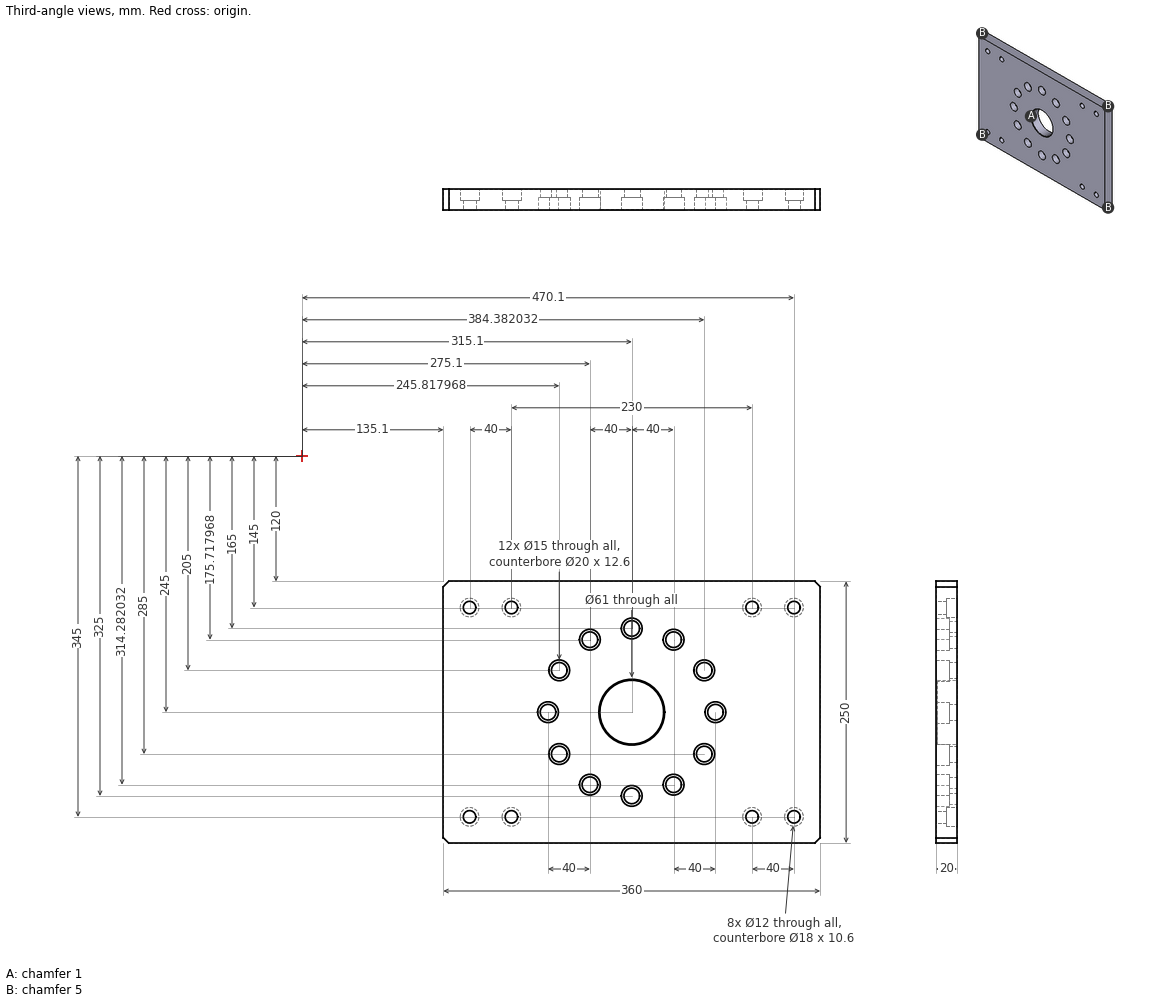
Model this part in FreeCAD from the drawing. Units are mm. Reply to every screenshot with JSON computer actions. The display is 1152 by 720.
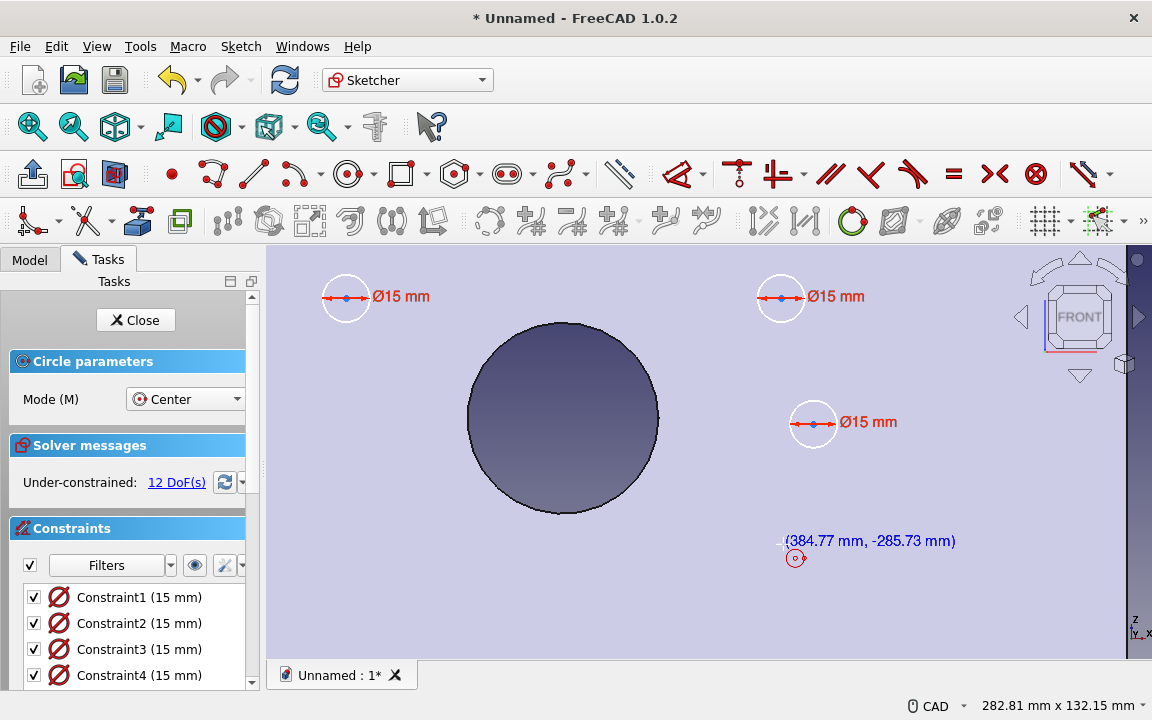
{"action": "scroll", "coordinate": [783, 544], "scroll_direction": "down", "scroll_amount": 7}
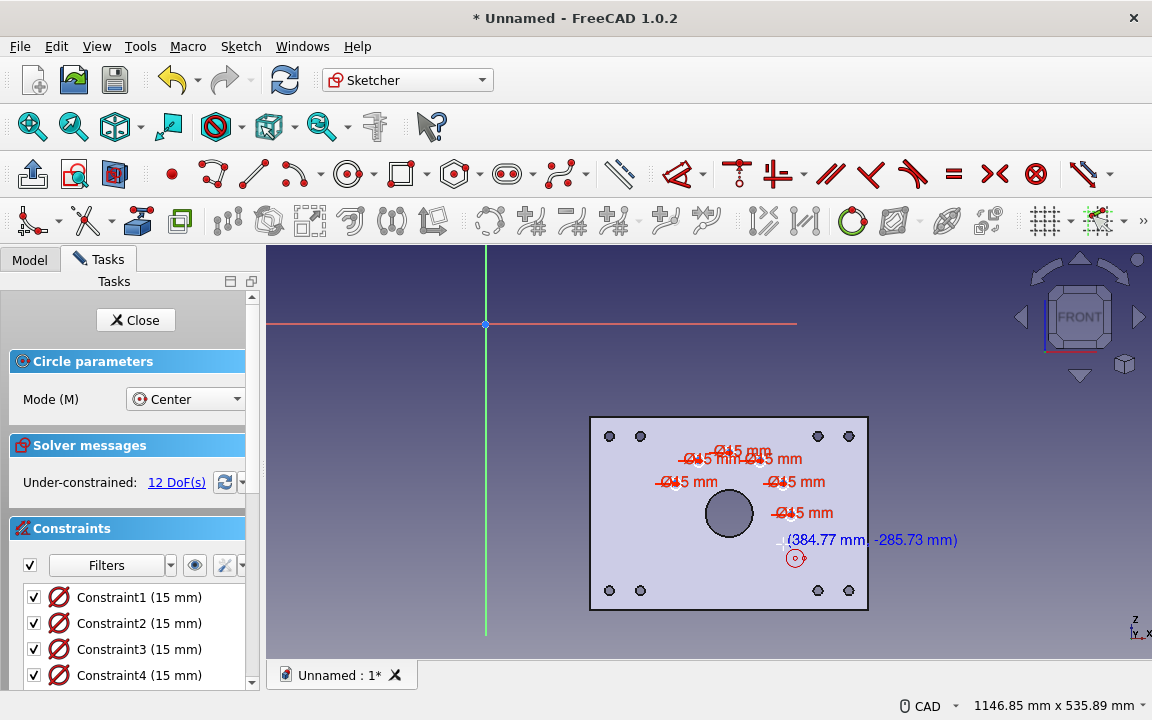
{"action": "left_click", "coordinate": [783, 544]}
{"action": "mouse_move", "coordinate": [787, 540]}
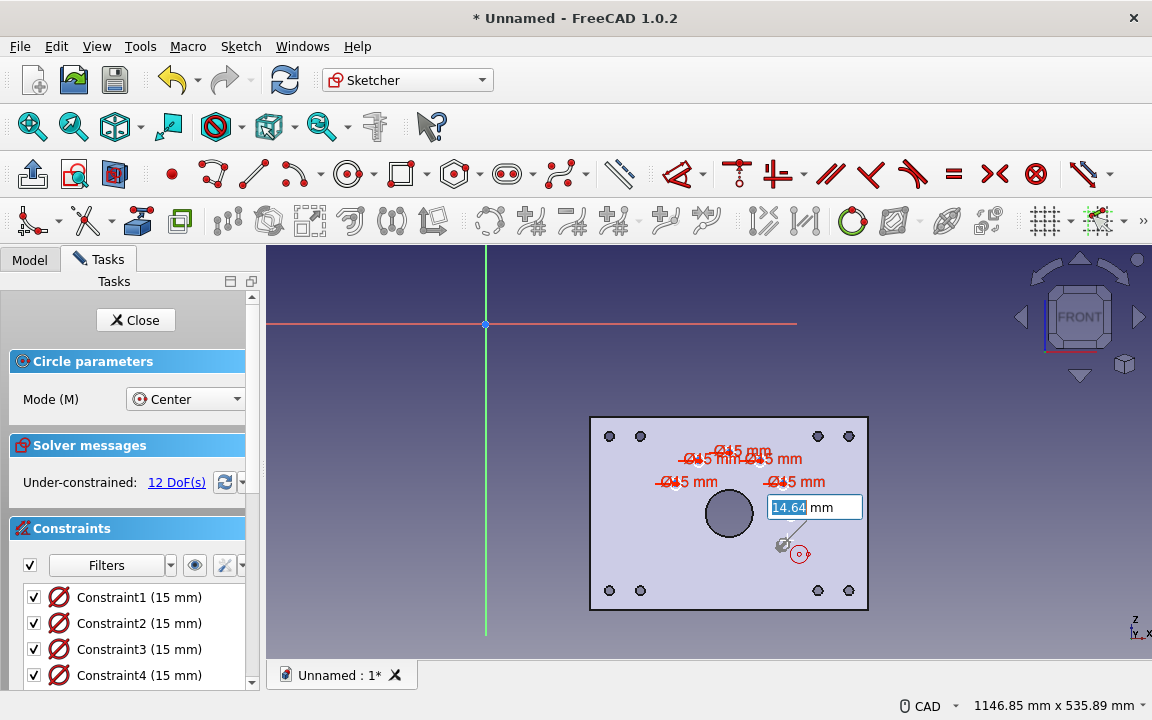
{"action": "type", "text": "15"}
{"action": "key", "text": "Return"}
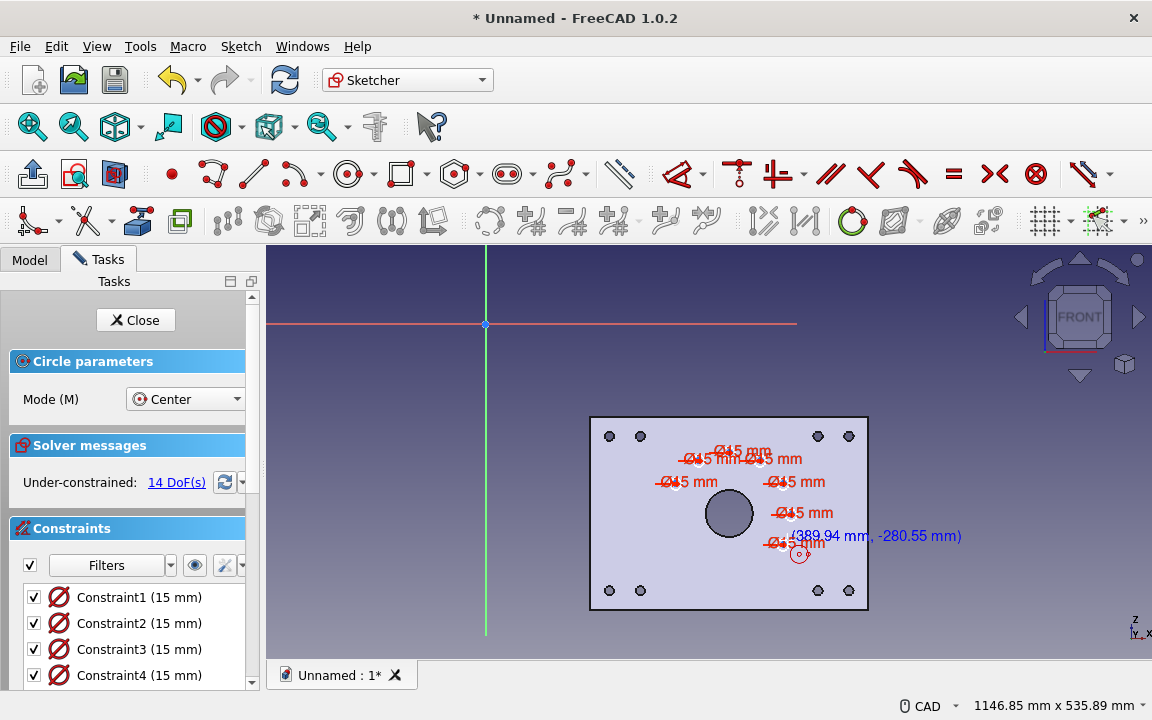
{"action": "scroll", "coordinate": [760, 567], "scroll_direction": "up", "scroll_amount": 7}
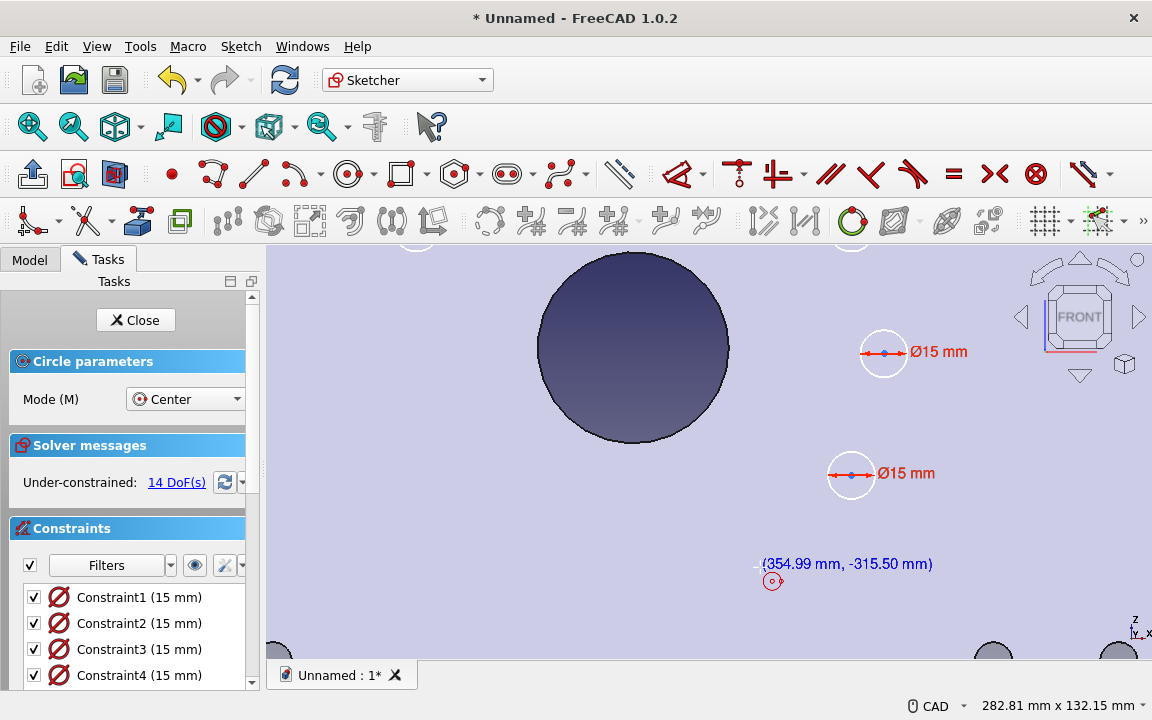
{"action": "scroll", "coordinate": [760, 567], "scroll_direction": "down", "scroll_amount": 7}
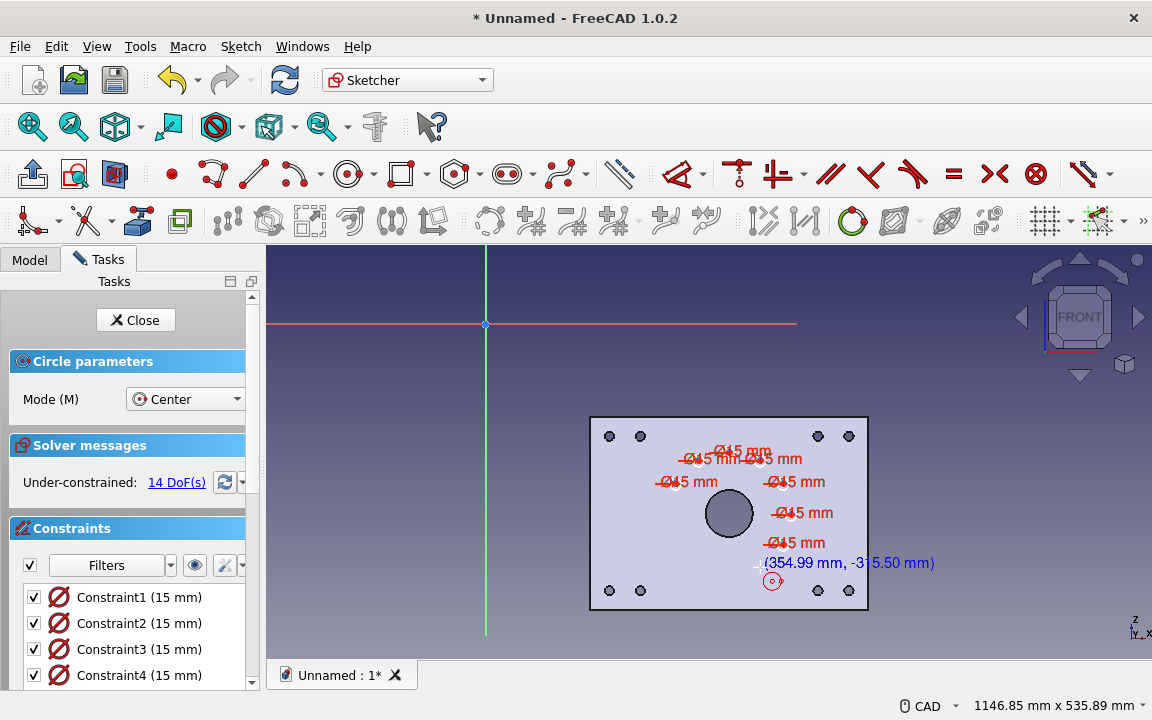
{"action": "left_click", "coordinate": [760, 567]}
{"action": "mouse_move", "coordinate": [764, 563]}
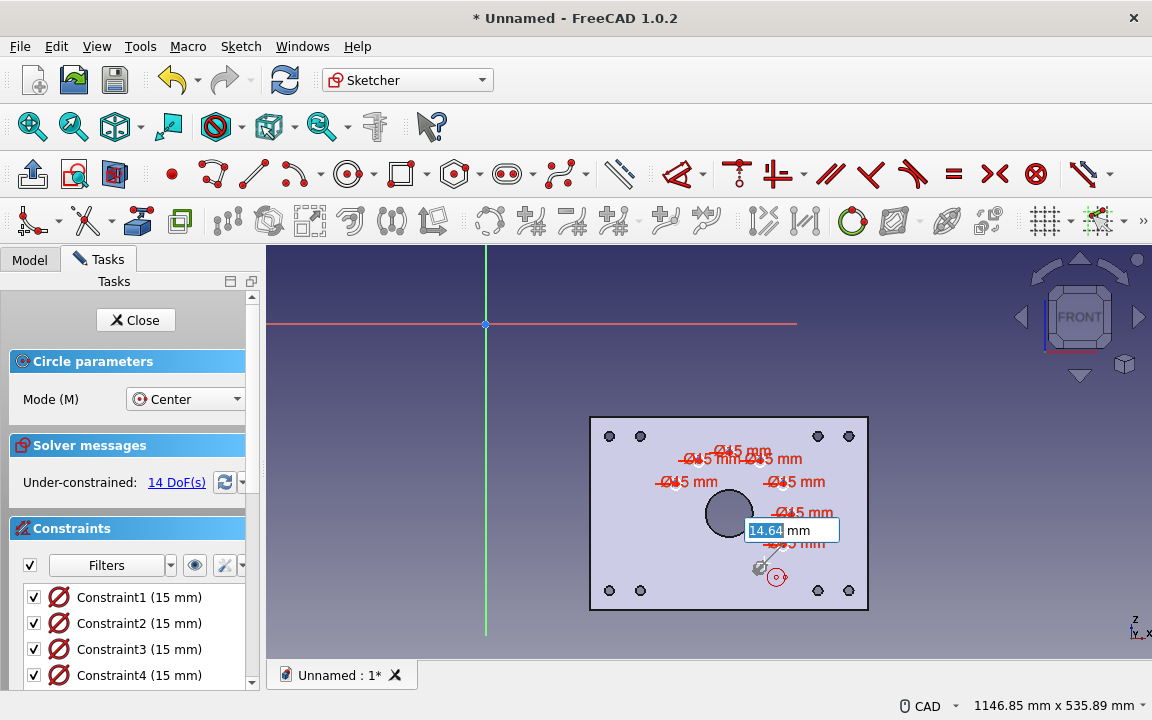
{"action": "type", "text": "15"}
{"action": "key", "text": "Return"}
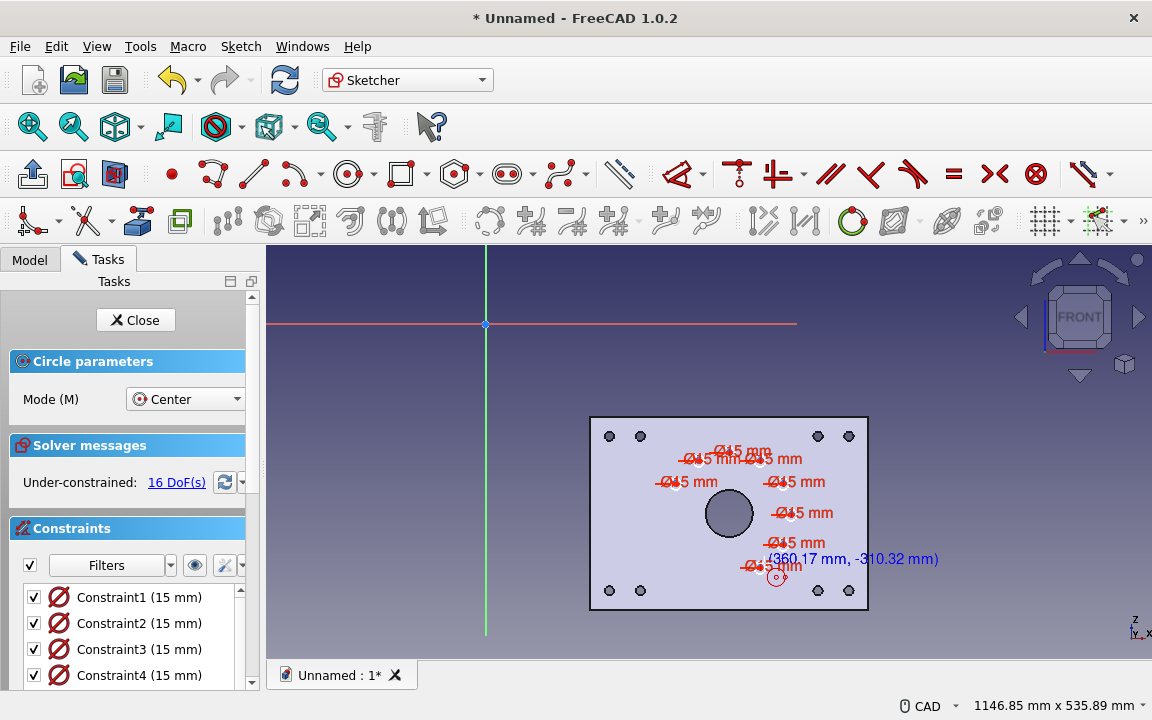
{"action": "scroll", "coordinate": [729, 575], "scroll_direction": "up", "scroll_amount": 7}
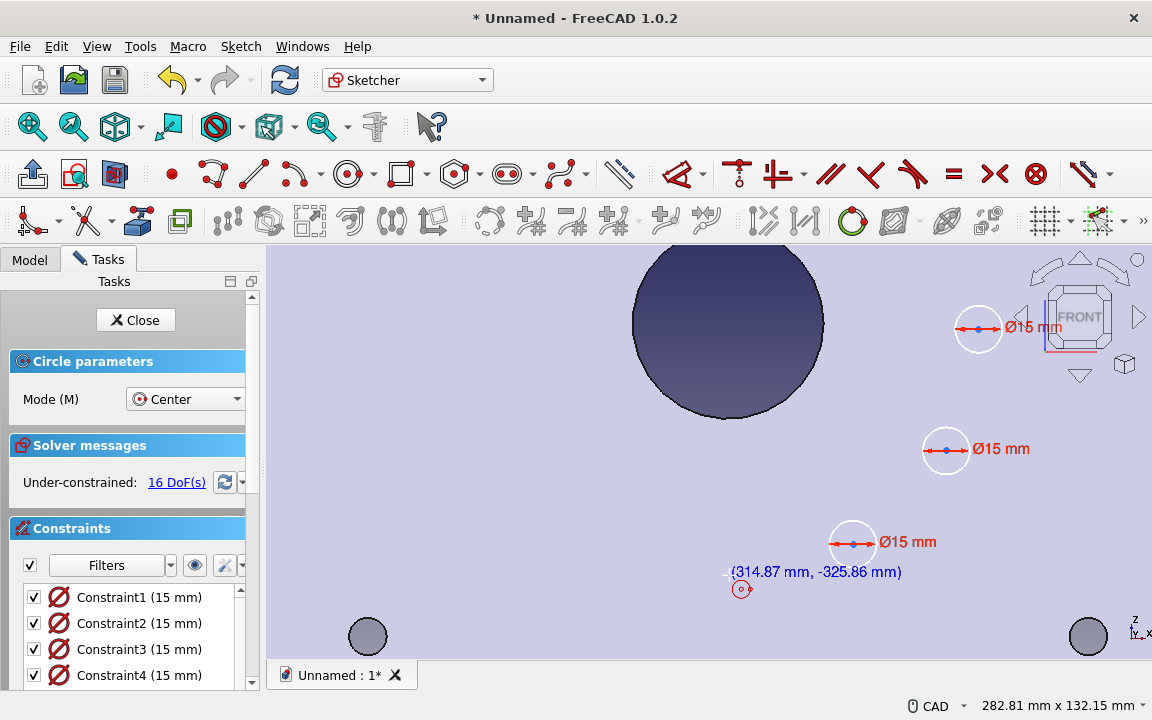
{"action": "scroll", "coordinate": [729, 575], "scroll_direction": "down", "scroll_amount": 7}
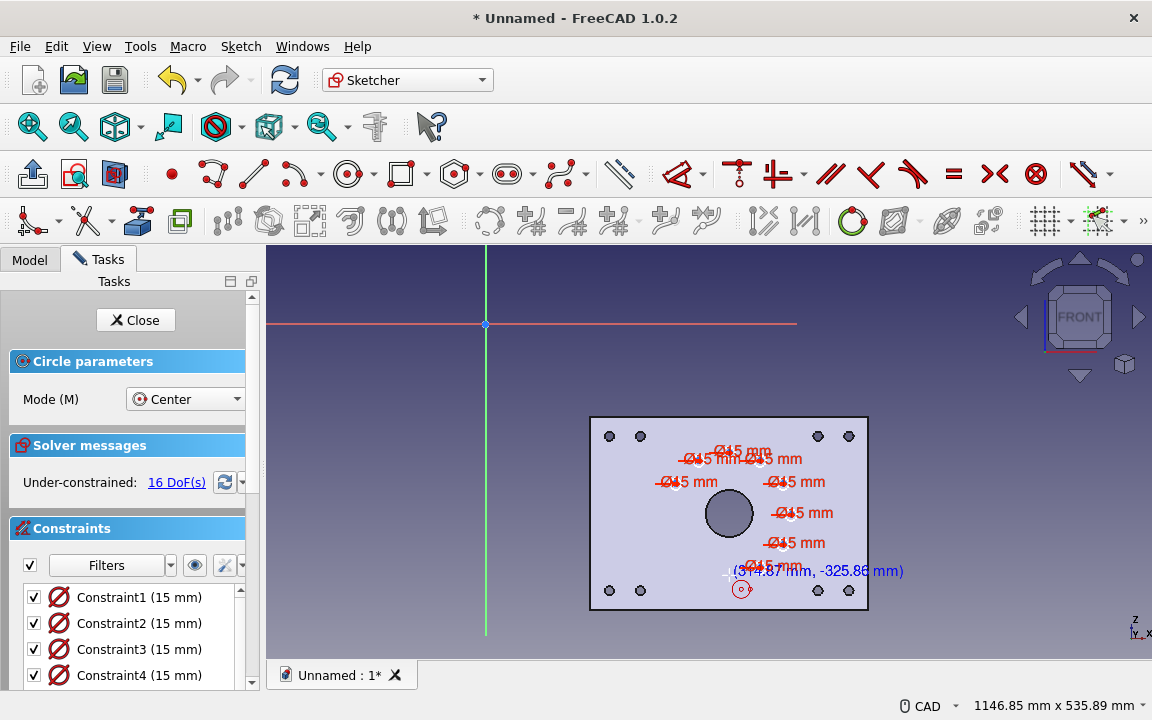
{"action": "left_click", "coordinate": [729, 575]}
{"action": "mouse_move", "coordinate": [733, 571]}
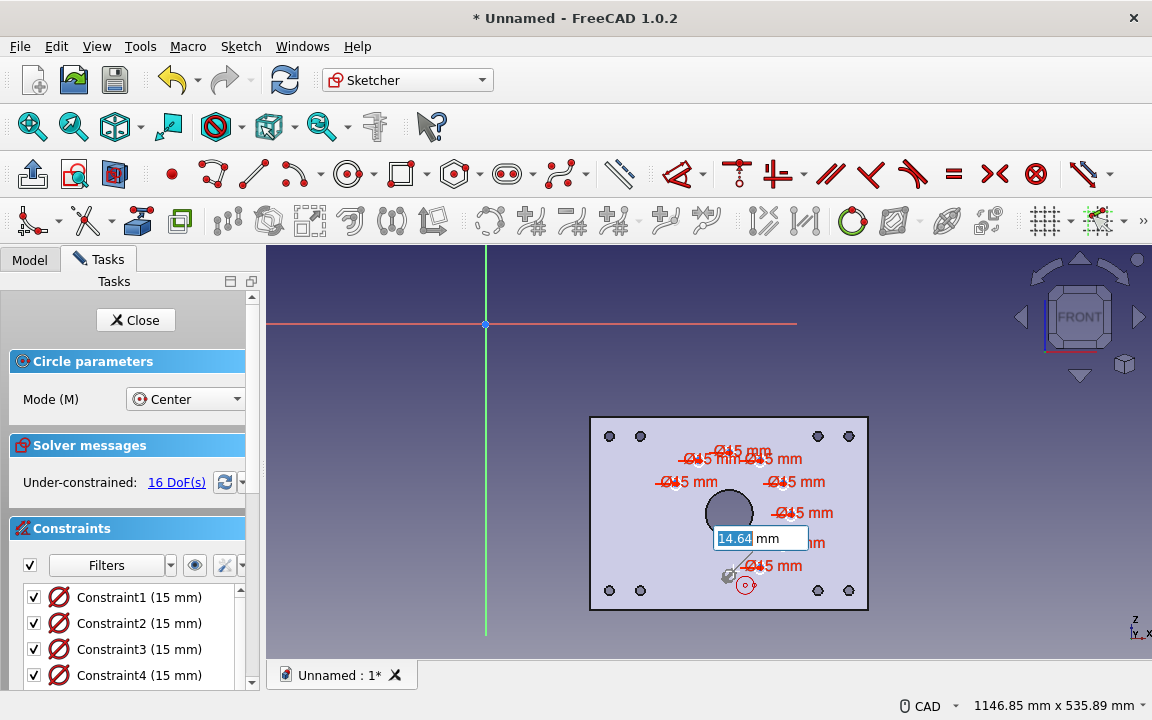
{"action": "type", "text": "15"}
{"action": "key", "text": "Return"}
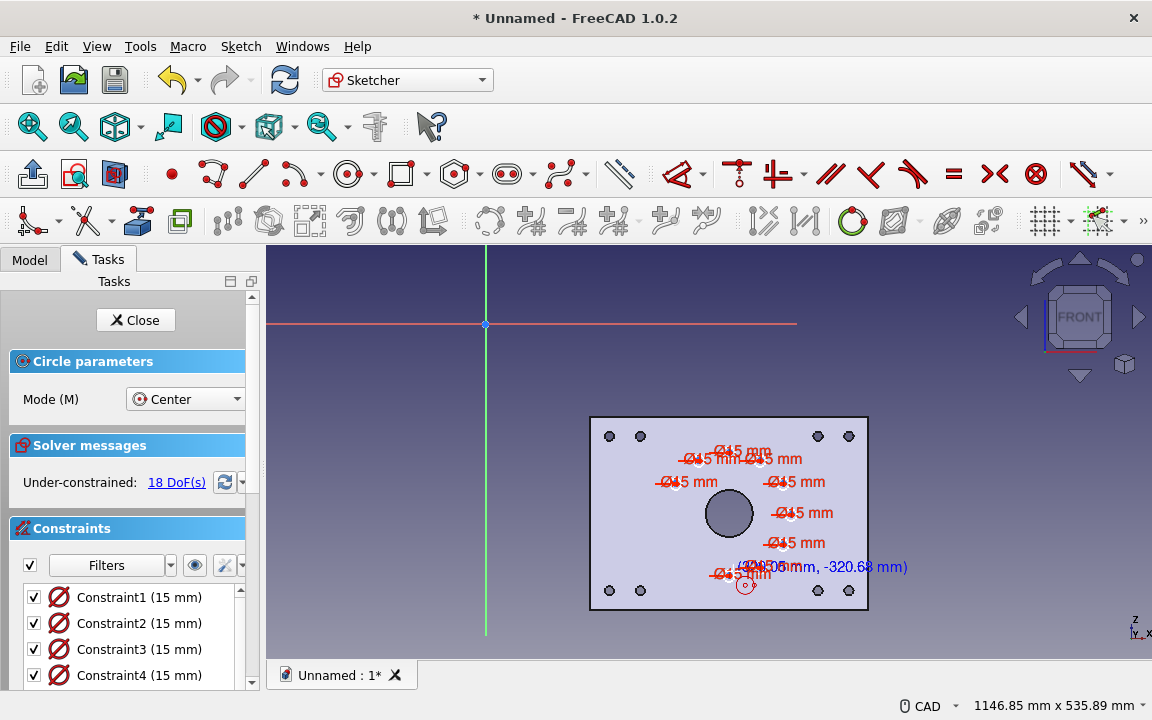
{"action": "scroll", "coordinate": [698, 567], "scroll_direction": "up", "scroll_amount": 7}